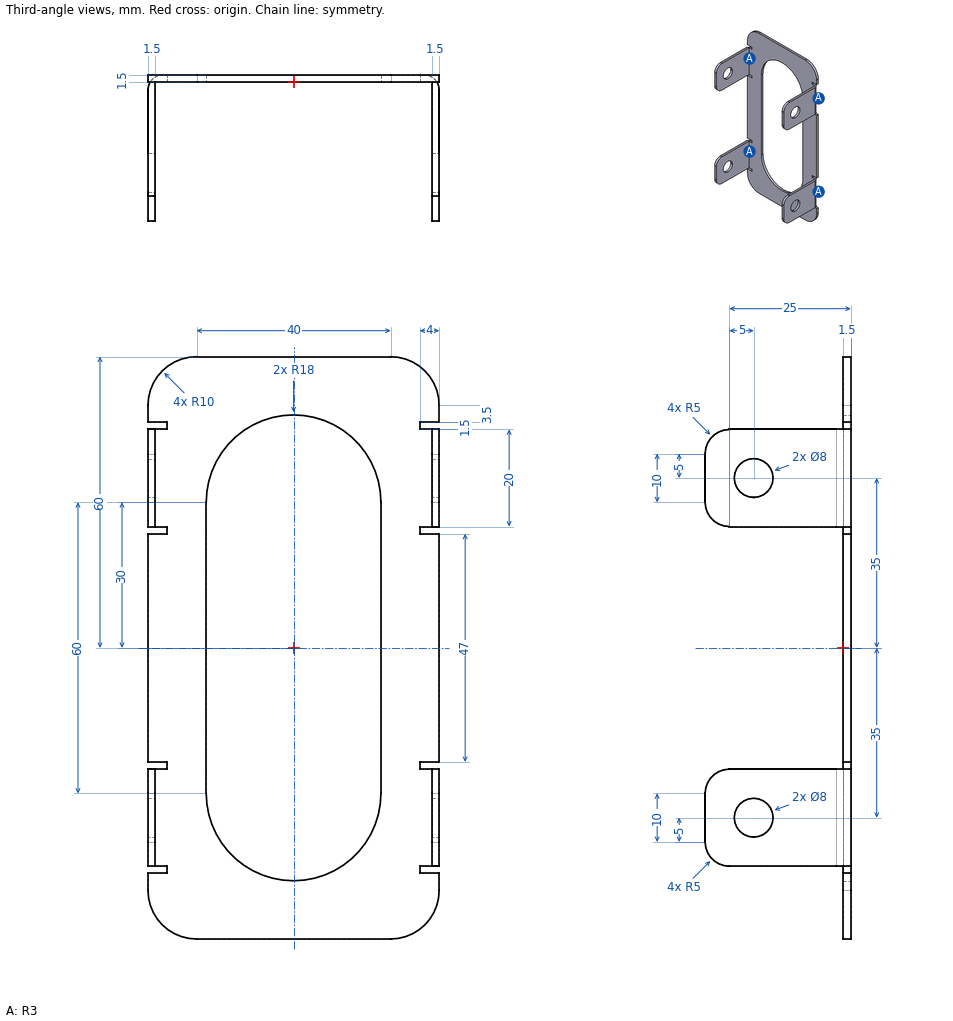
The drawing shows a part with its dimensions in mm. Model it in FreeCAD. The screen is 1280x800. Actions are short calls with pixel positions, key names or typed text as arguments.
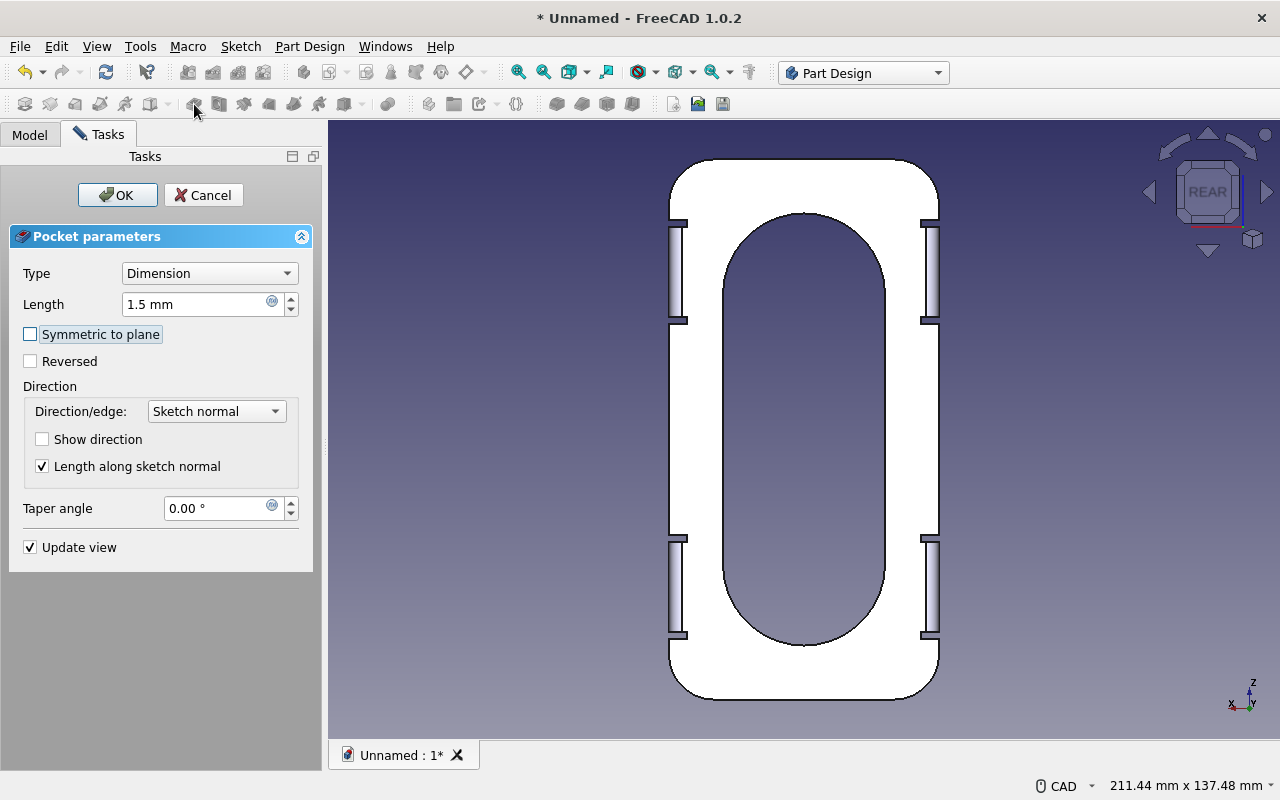
click(118, 195)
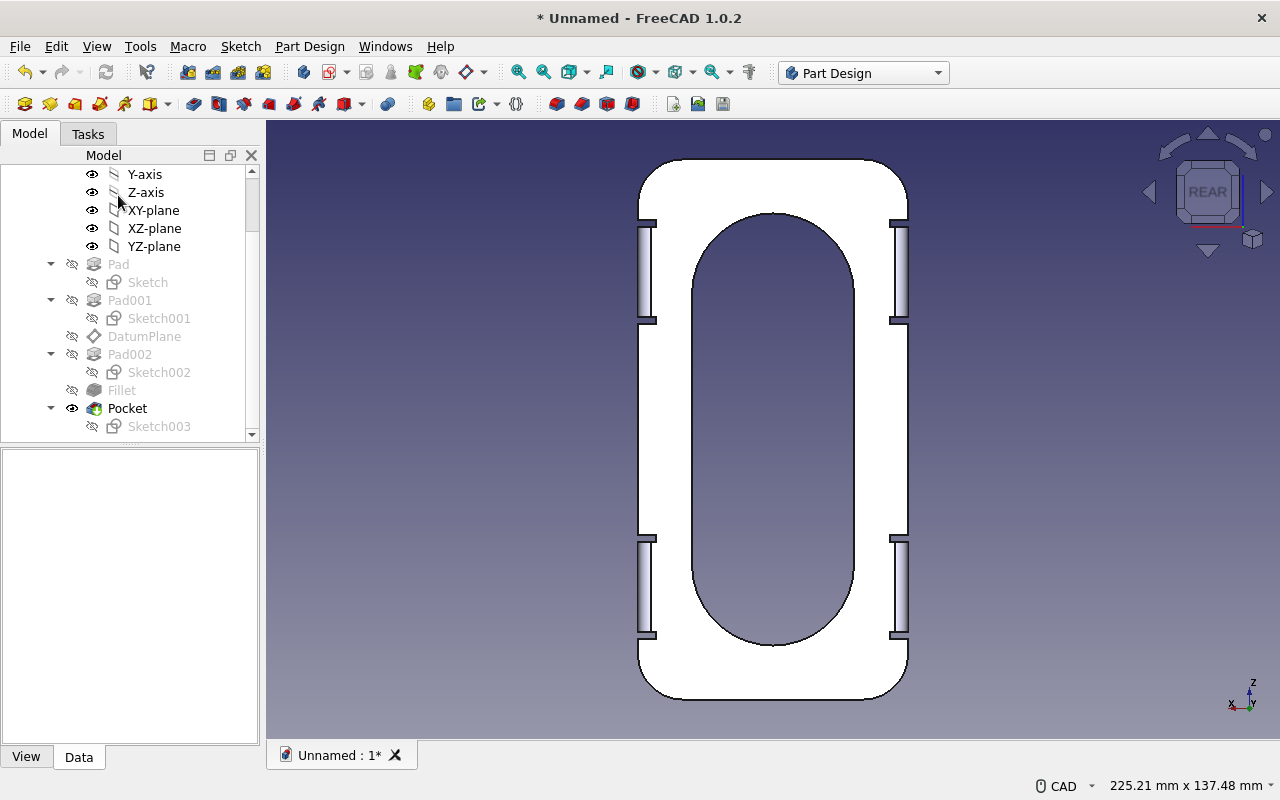
key(0)